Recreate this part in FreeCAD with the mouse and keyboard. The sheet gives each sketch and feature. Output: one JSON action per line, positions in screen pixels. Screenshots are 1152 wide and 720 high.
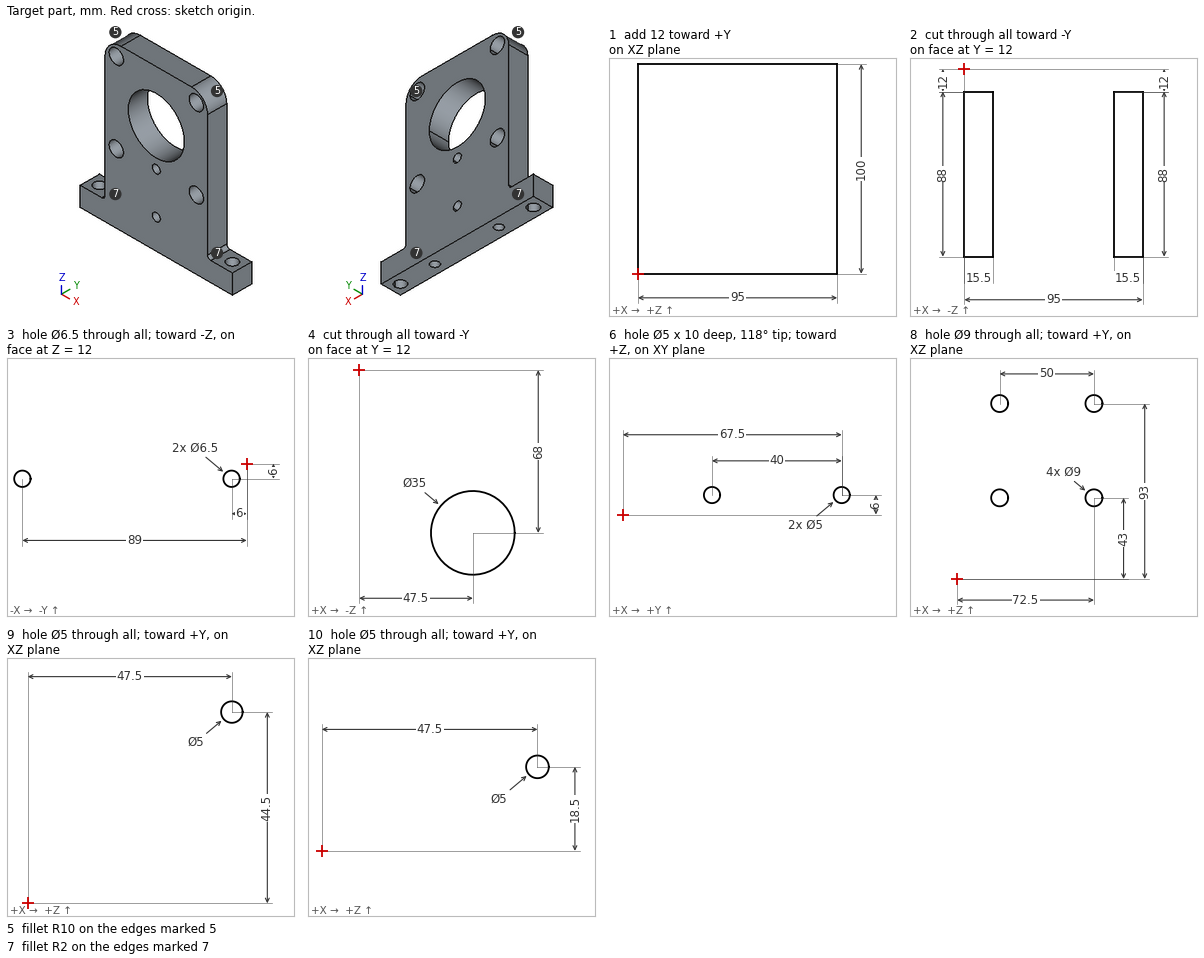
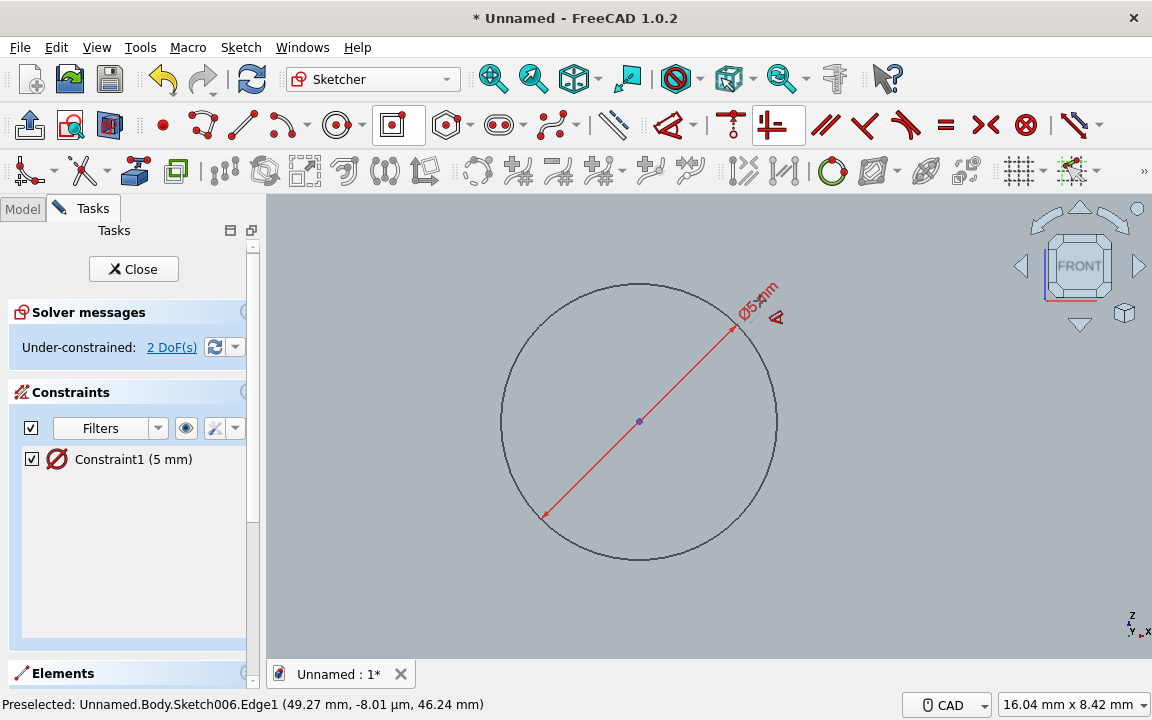
{"action": "left_click", "coordinate": [639, 422]}
{"action": "left_click", "coordinate": [467, 388]}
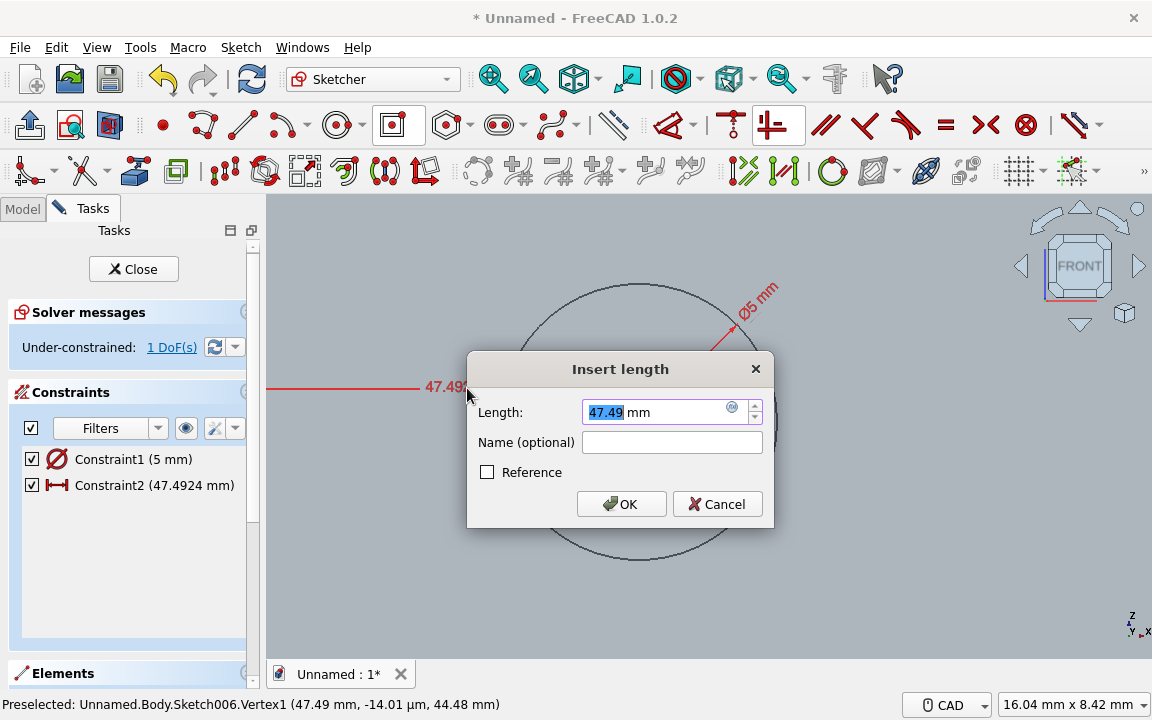
{"action": "type", "text": "47.5"}
{"action": "key", "text": "Return"}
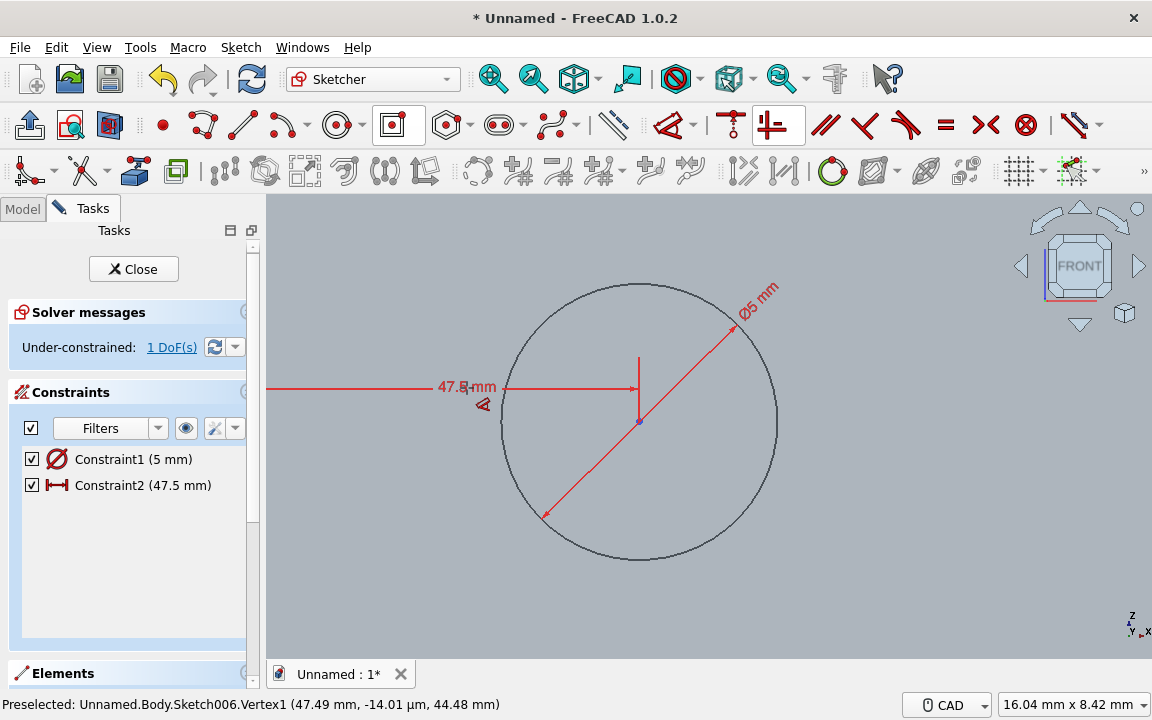
{"action": "left_click", "coordinate": [639, 422]}
{"action": "left_click", "coordinate": [673, 526]}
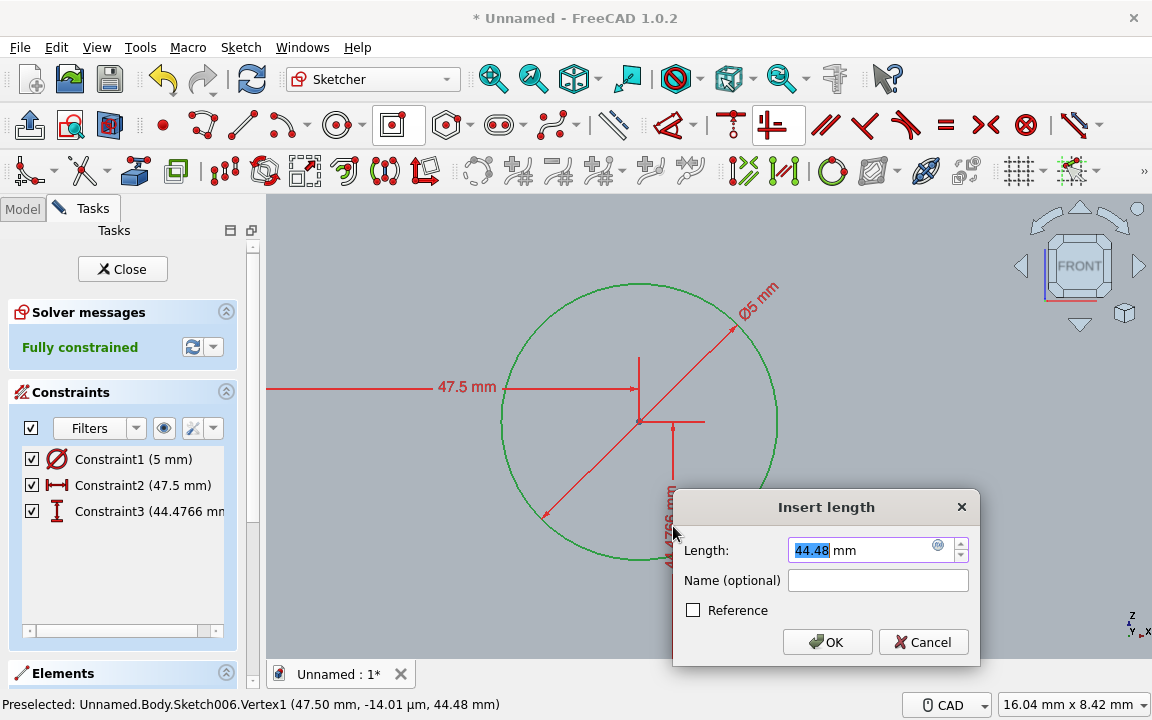
{"action": "type", "text": "44.5"}
{"action": "key", "text": "Return"}
{"action": "key", "text": "Escape"}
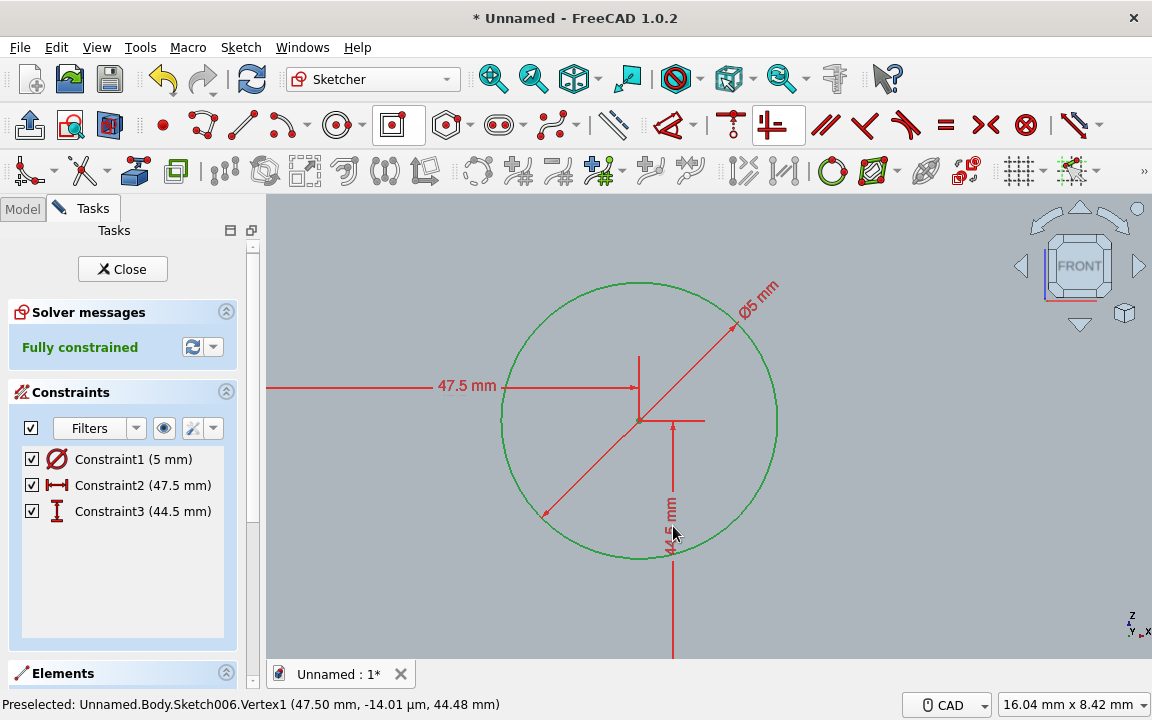
{"action": "left_click", "coordinate": [123, 269]}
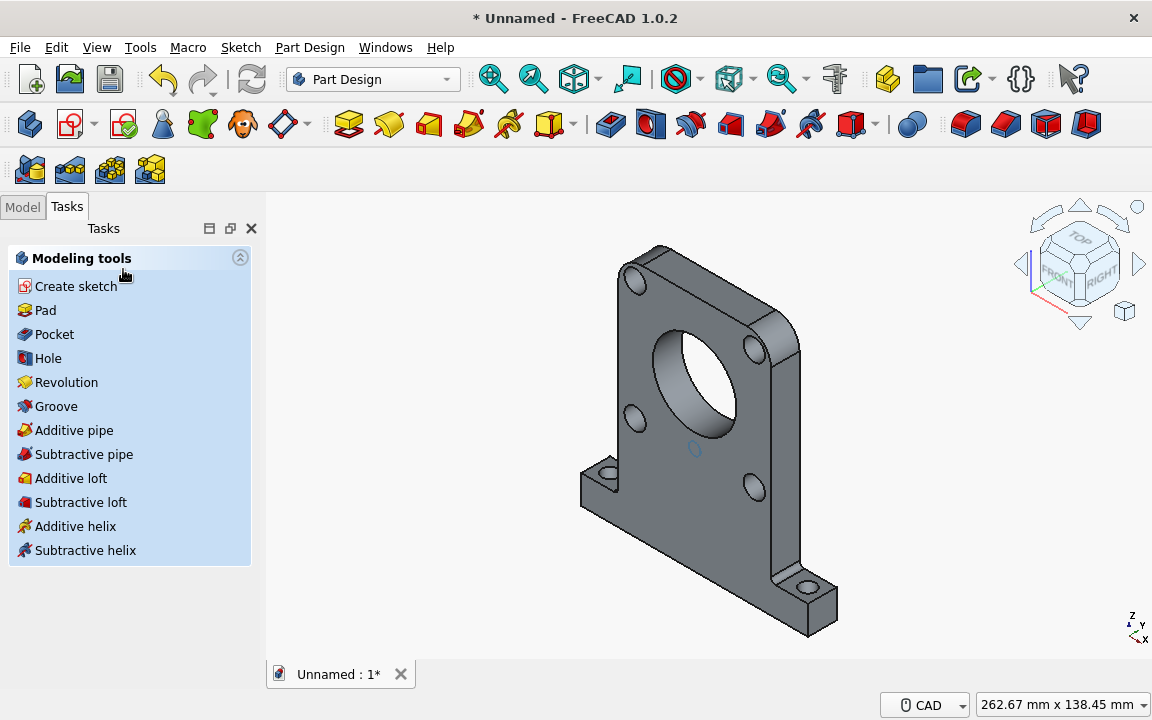
{"action": "left_click", "coordinate": [652, 124]}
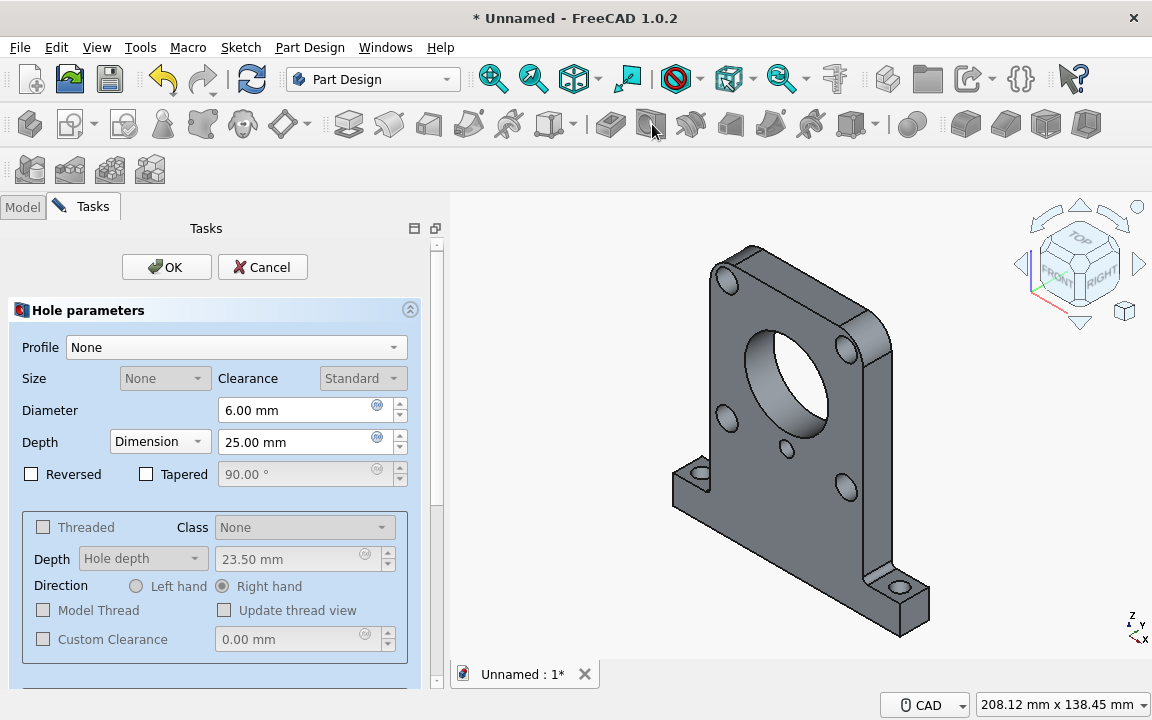
{"action": "triple_click", "coordinate": [305, 410]}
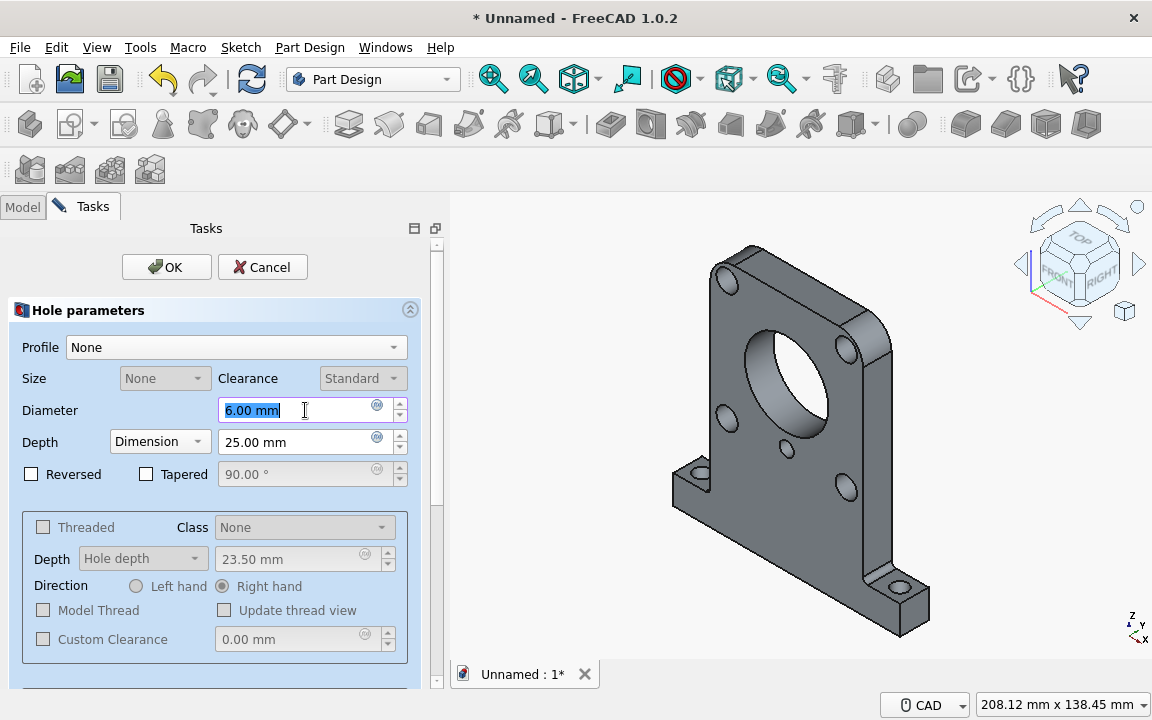
{"action": "type", "text": "5"}
{"action": "key", "text": "Tab"}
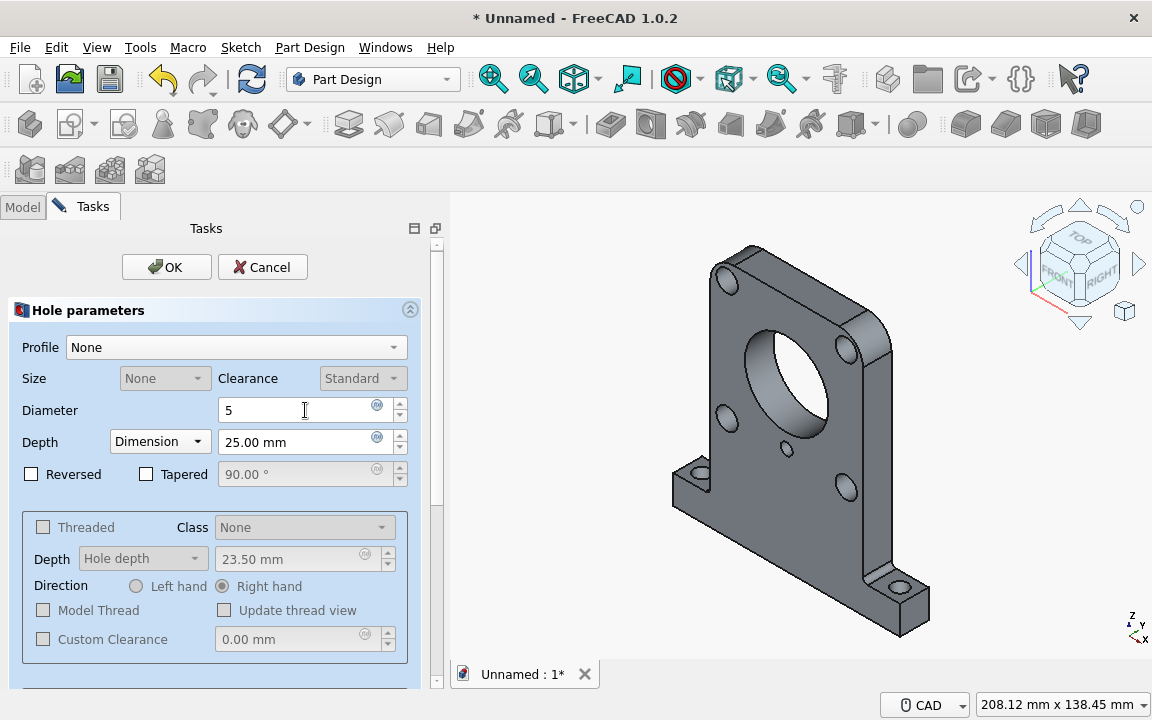
{"action": "left_click", "coordinate": [161, 442]}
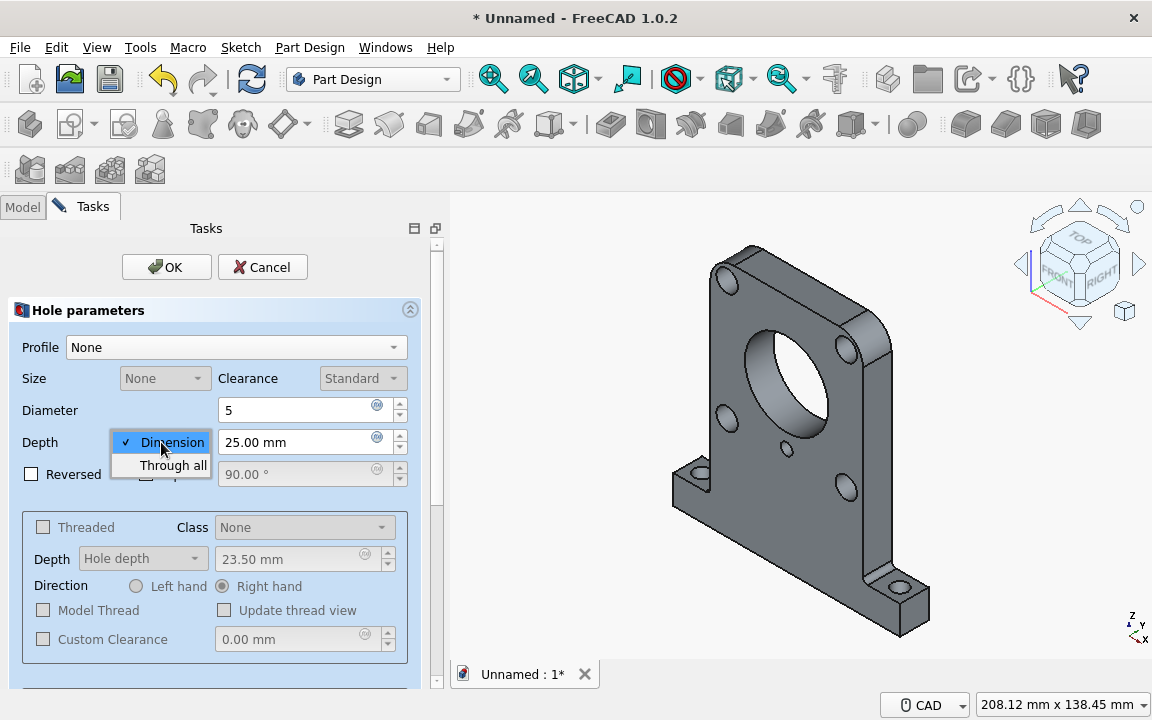
{"action": "left_click", "coordinate": [160, 466]}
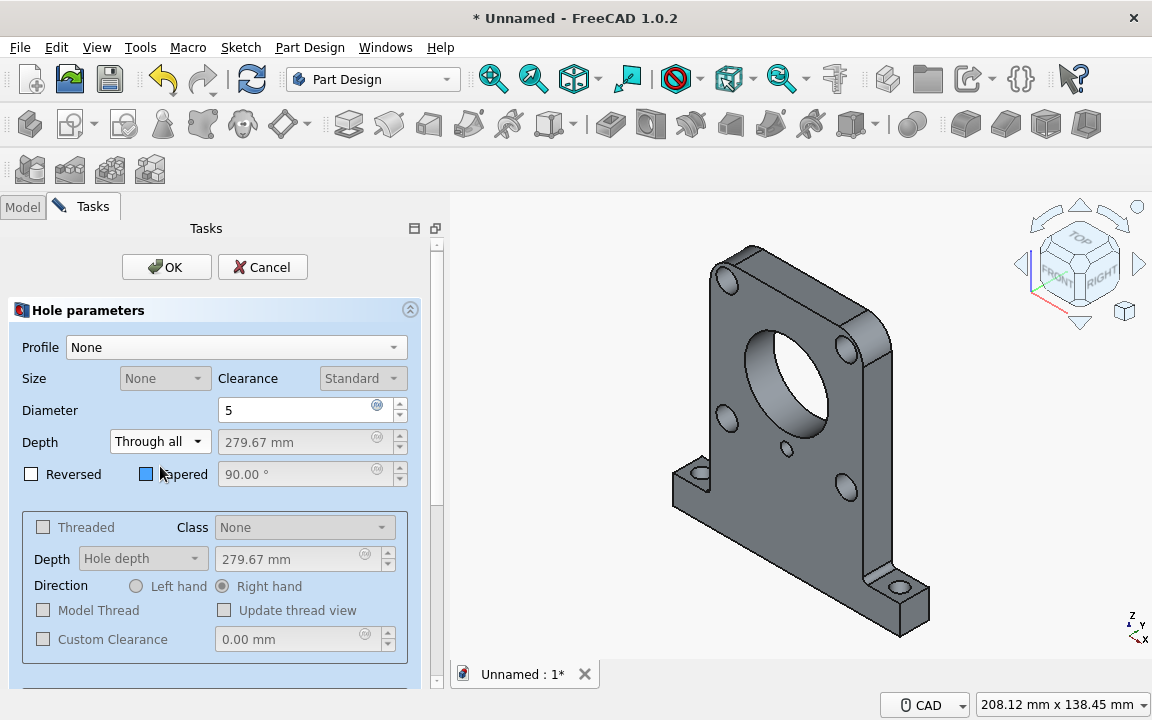
{"action": "left_click", "coordinate": [167, 267]}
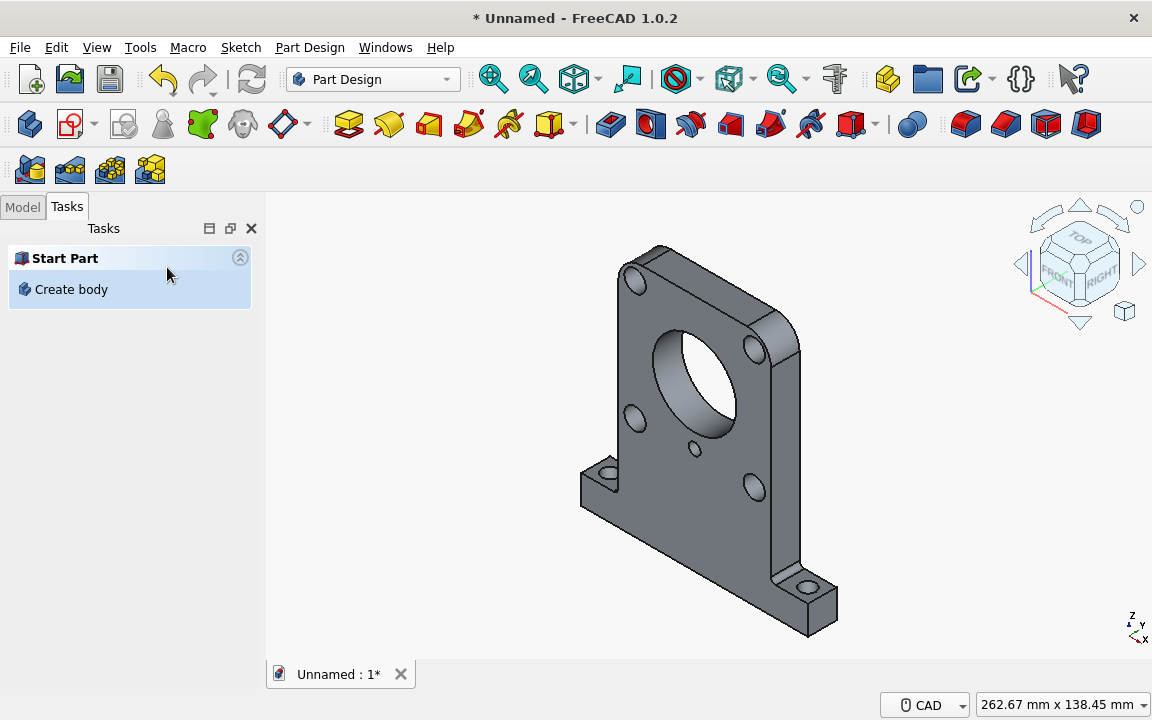
{"action": "left_click", "coordinate": [70, 124]}